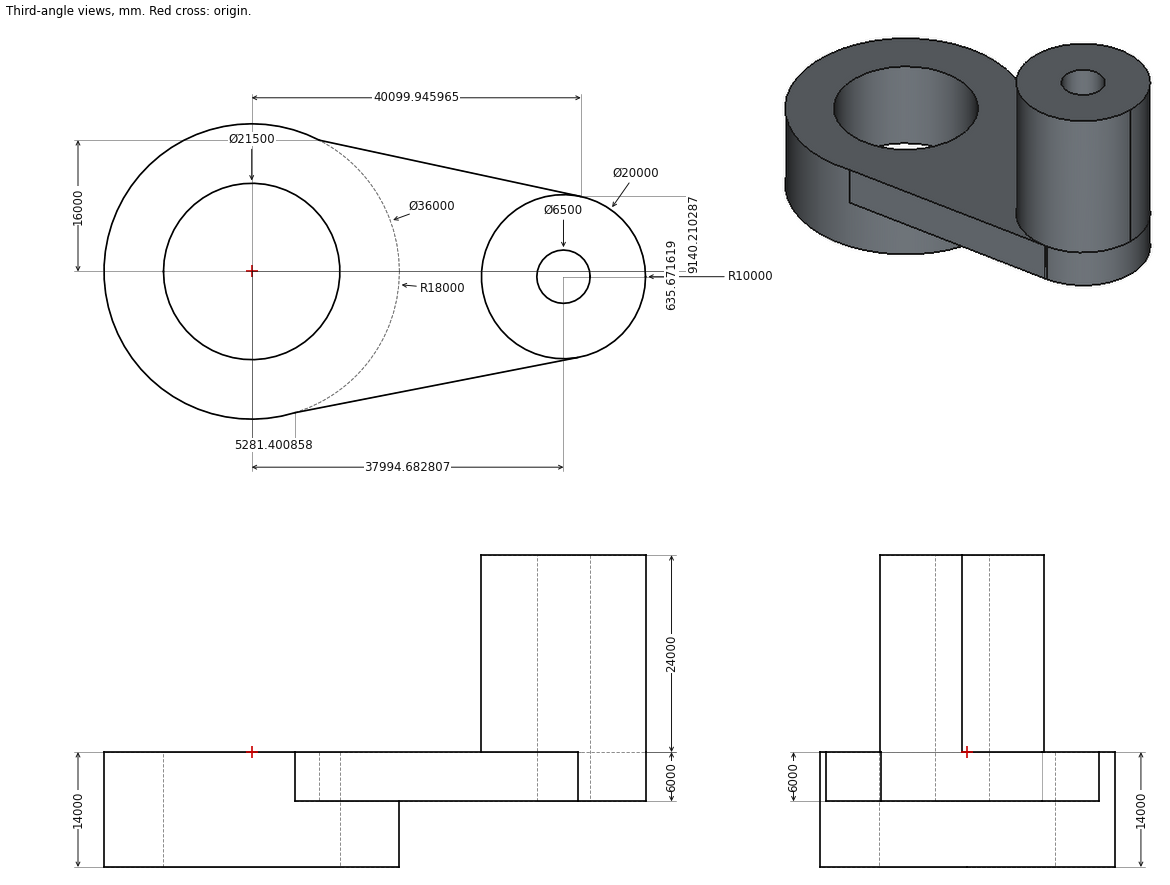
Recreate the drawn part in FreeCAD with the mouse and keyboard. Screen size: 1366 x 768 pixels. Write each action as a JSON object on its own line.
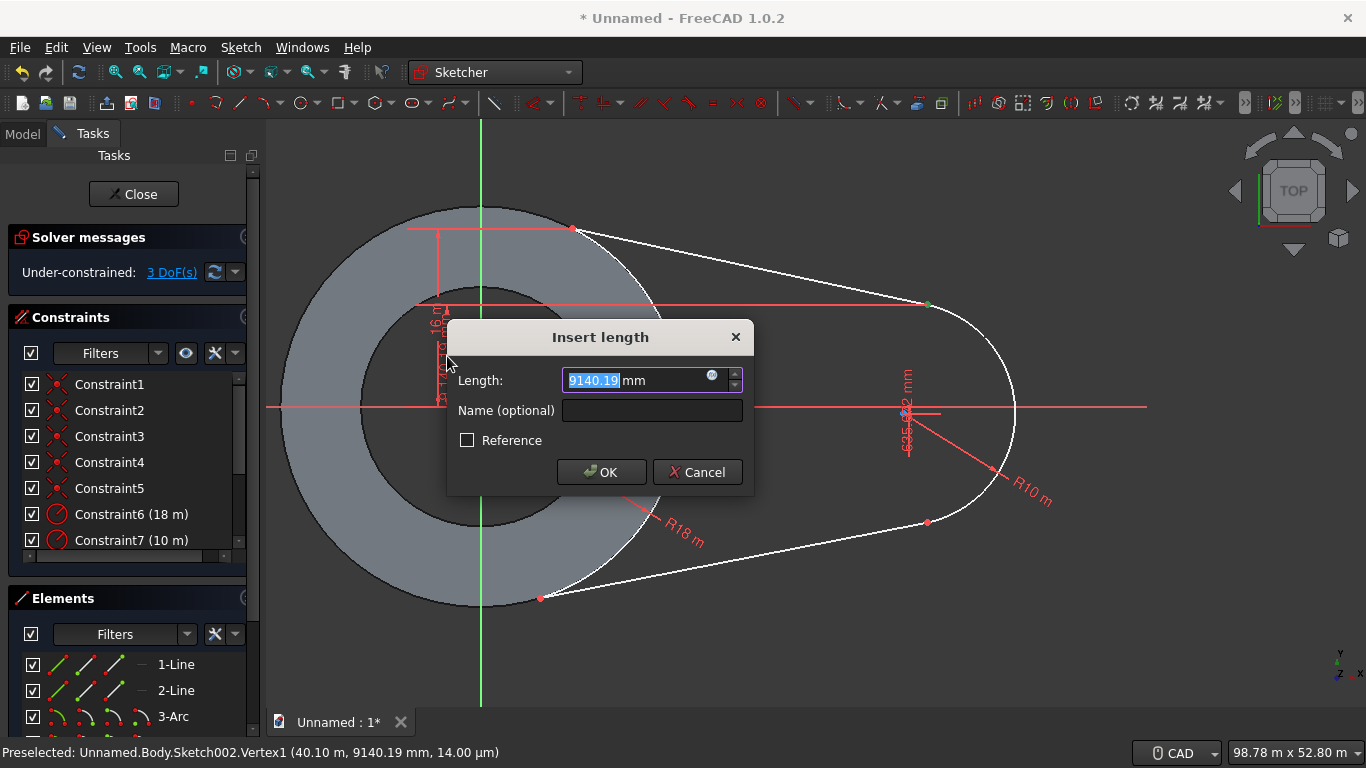
{"action": "type", "text": "9140.210287"}
{"action": "key", "text": "Return"}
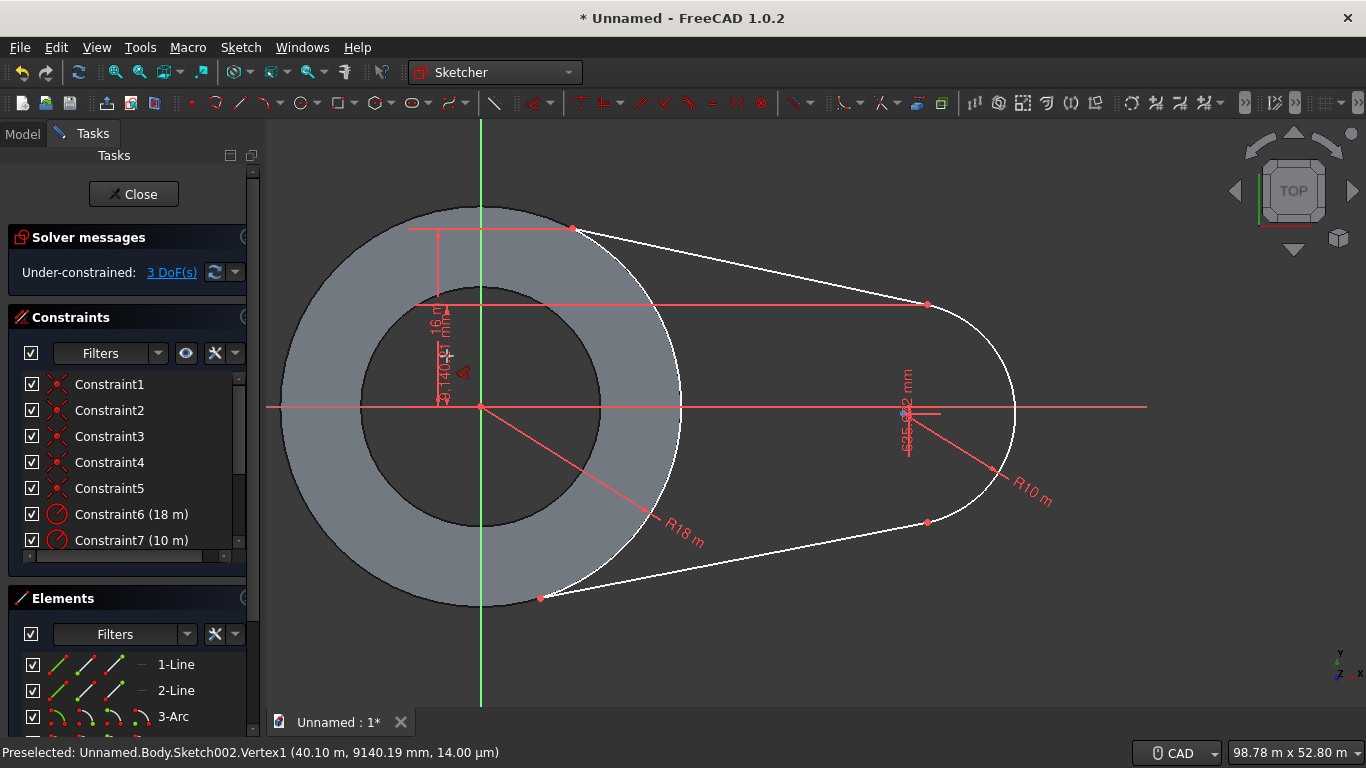
{"action": "left_click", "coordinate": [540, 598]}
{"action": "left_click", "coordinate": [510, 632]}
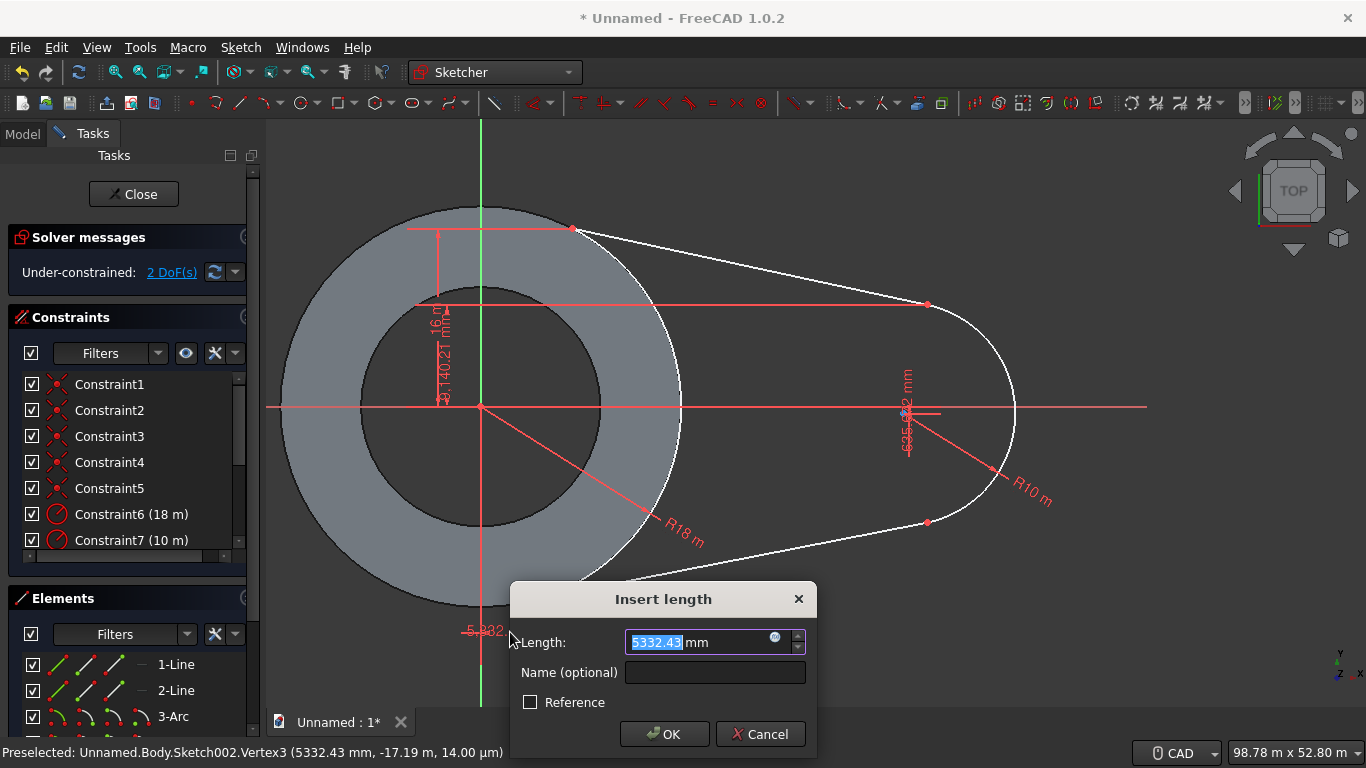
{"action": "type", "text": "5281.400858"}
{"action": "key", "text": "Return"}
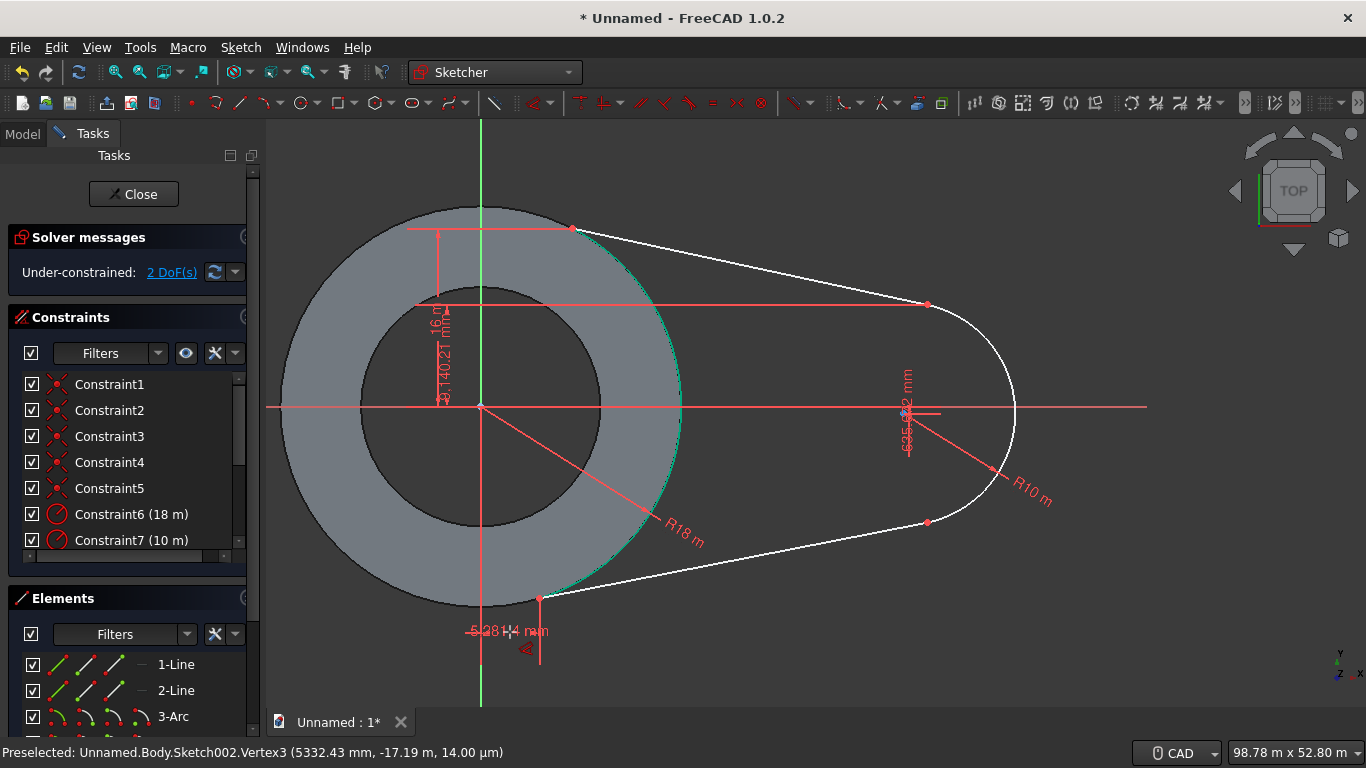
{"action": "left_click", "coordinate": [927, 305]}
{"action": "left_click", "coordinate": [704, 271]}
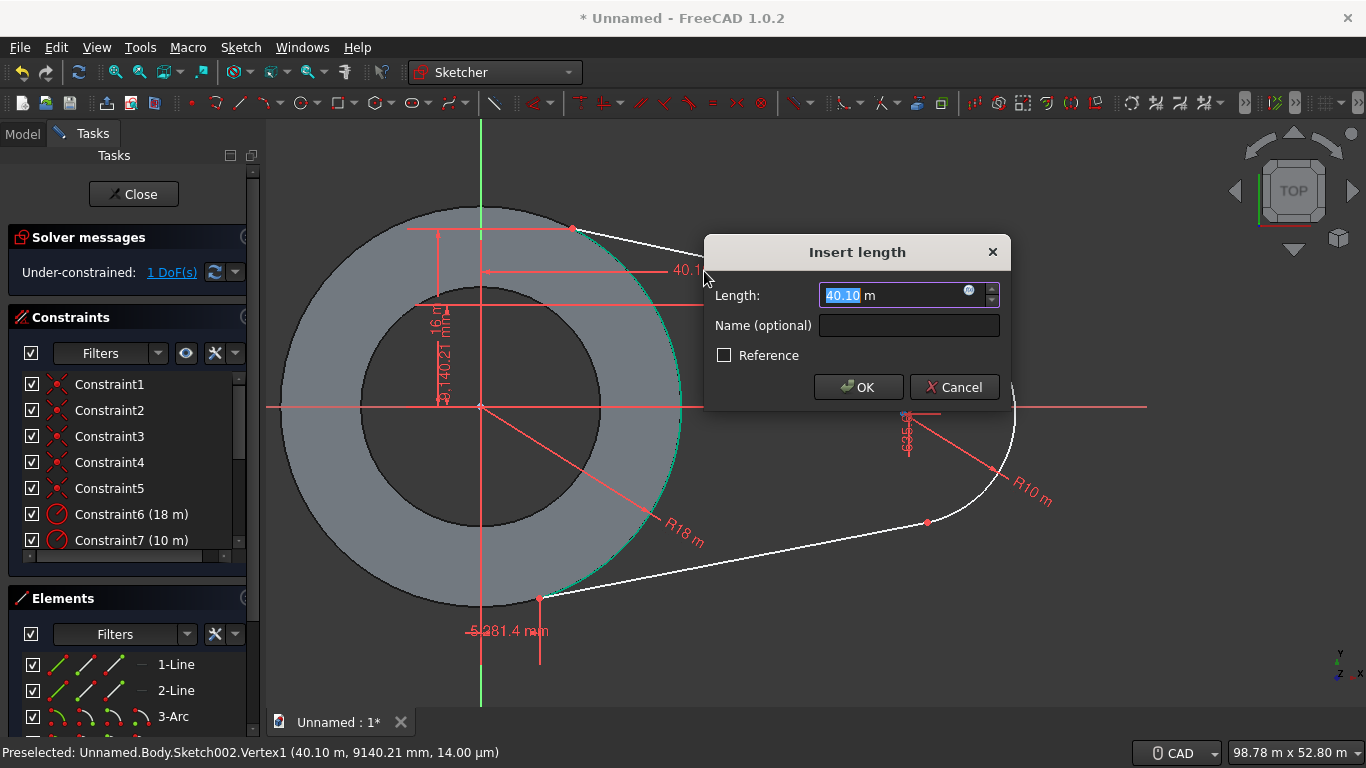
{"action": "key", "text": "ctrl+a"}
{"action": "type", "text": "40099.945965 mm"}
{"action": "key", "text": "Return"}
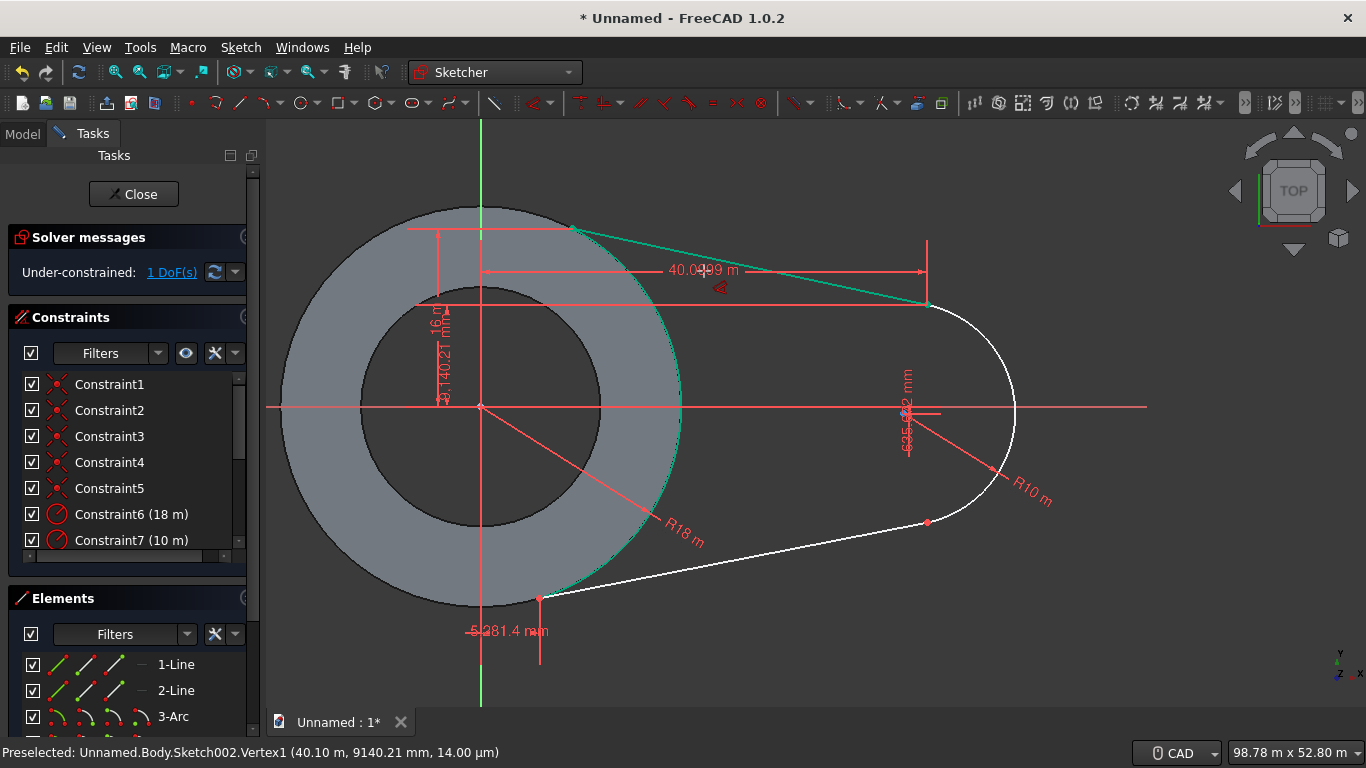
{"action": "left_click", "coordinate": [927, 523]}
{"action": "left_click", "coordinate": [548, 557]}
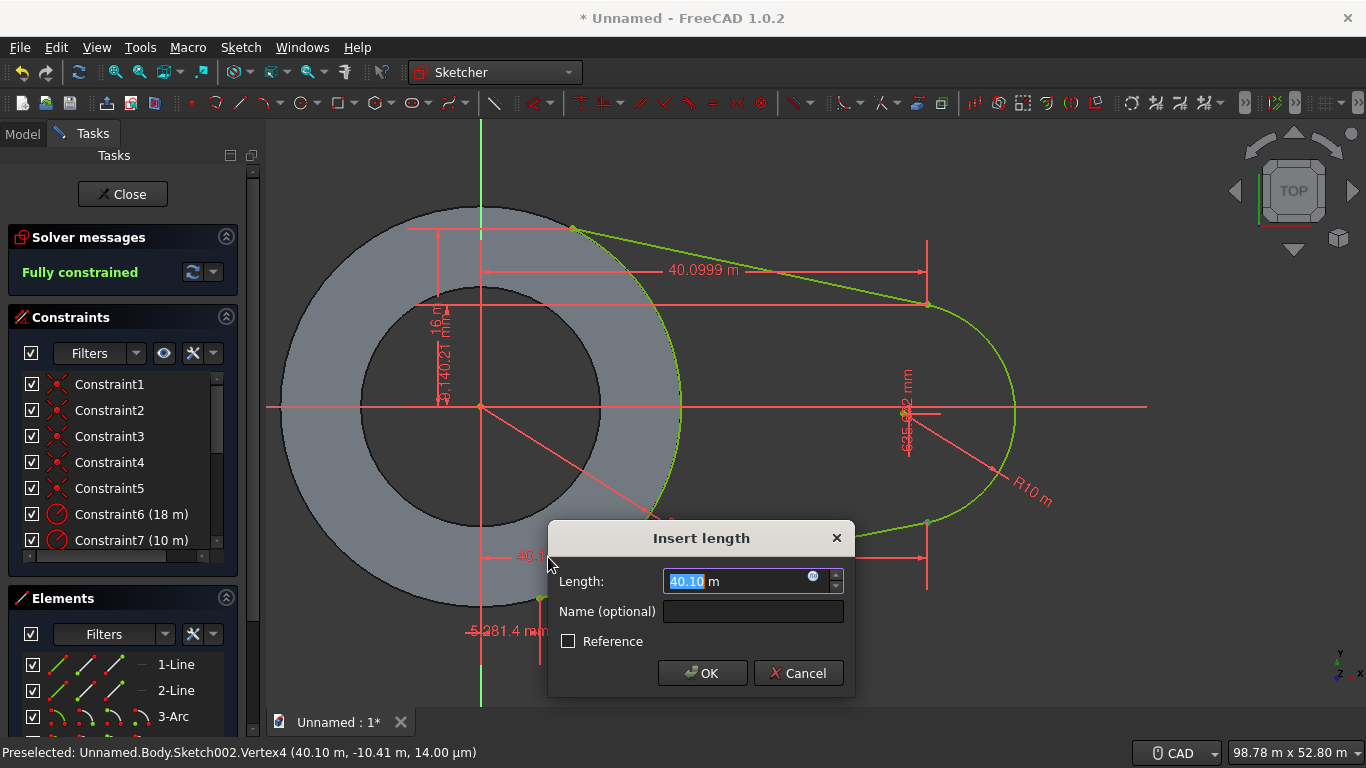
{"action": "key", "text": "ctrl+a"}
{"action": "type", "text": "40099.945965 mm"}
{"action": "key", "text": "Return"}
{"action": "key", "text": "Escape"}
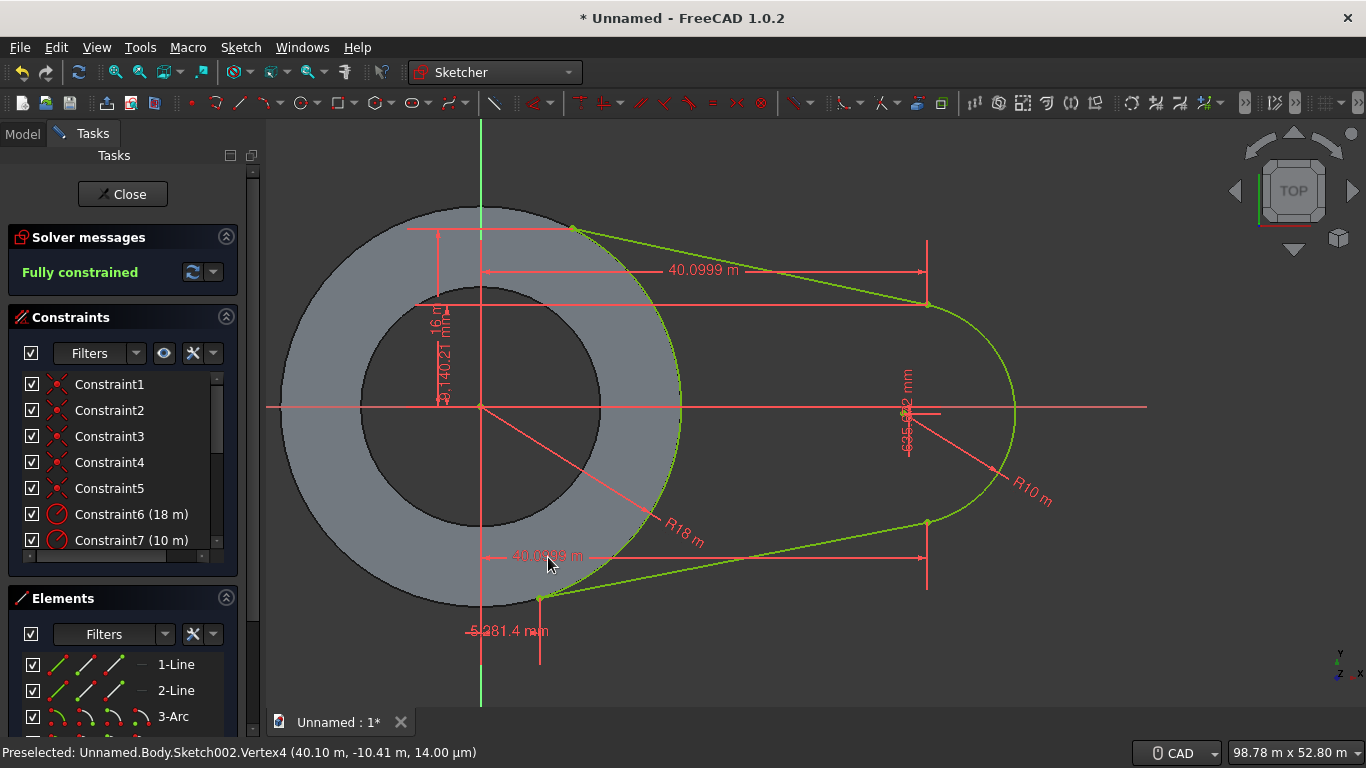
{"action": "left_click", "coordinate": [123, 194]}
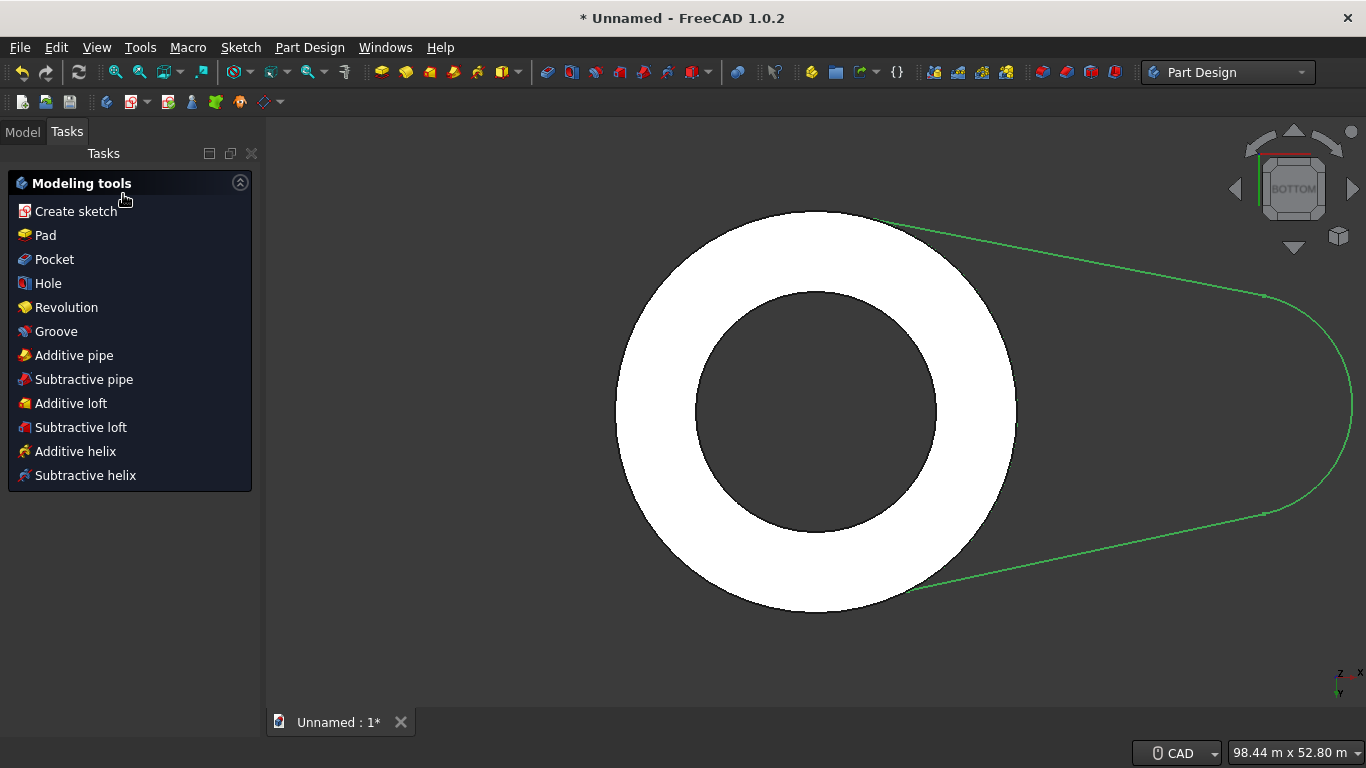
{"action": "left_click", "coordinate": [382, 72]}